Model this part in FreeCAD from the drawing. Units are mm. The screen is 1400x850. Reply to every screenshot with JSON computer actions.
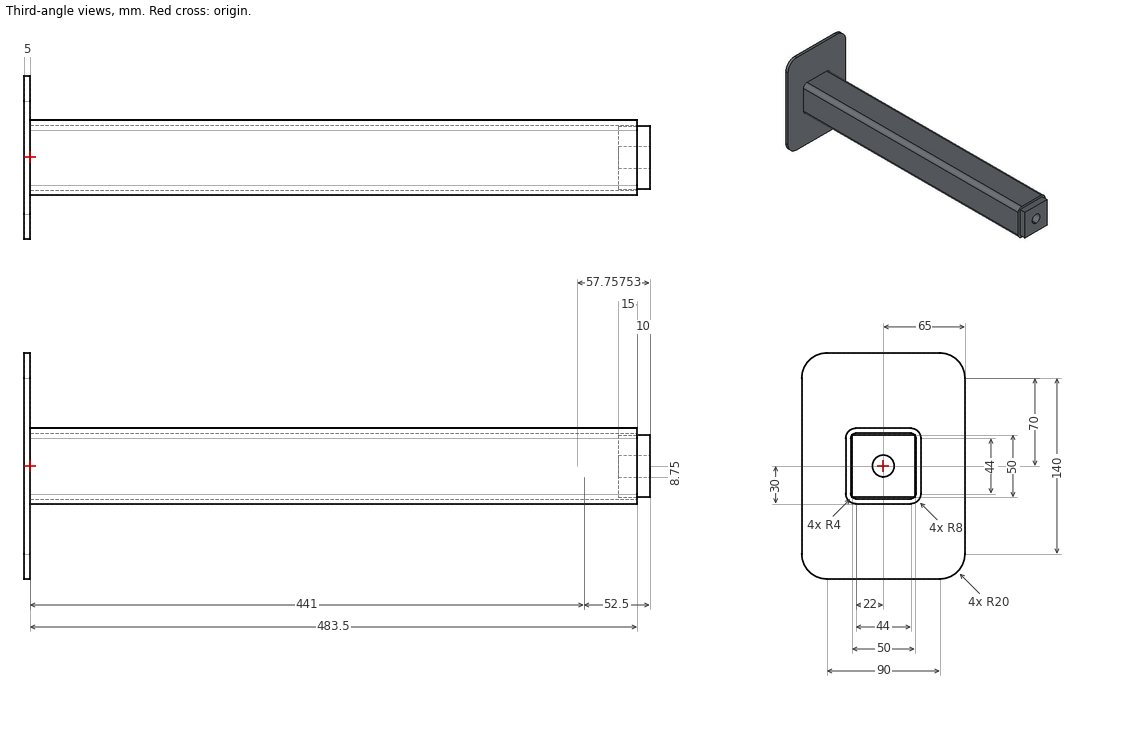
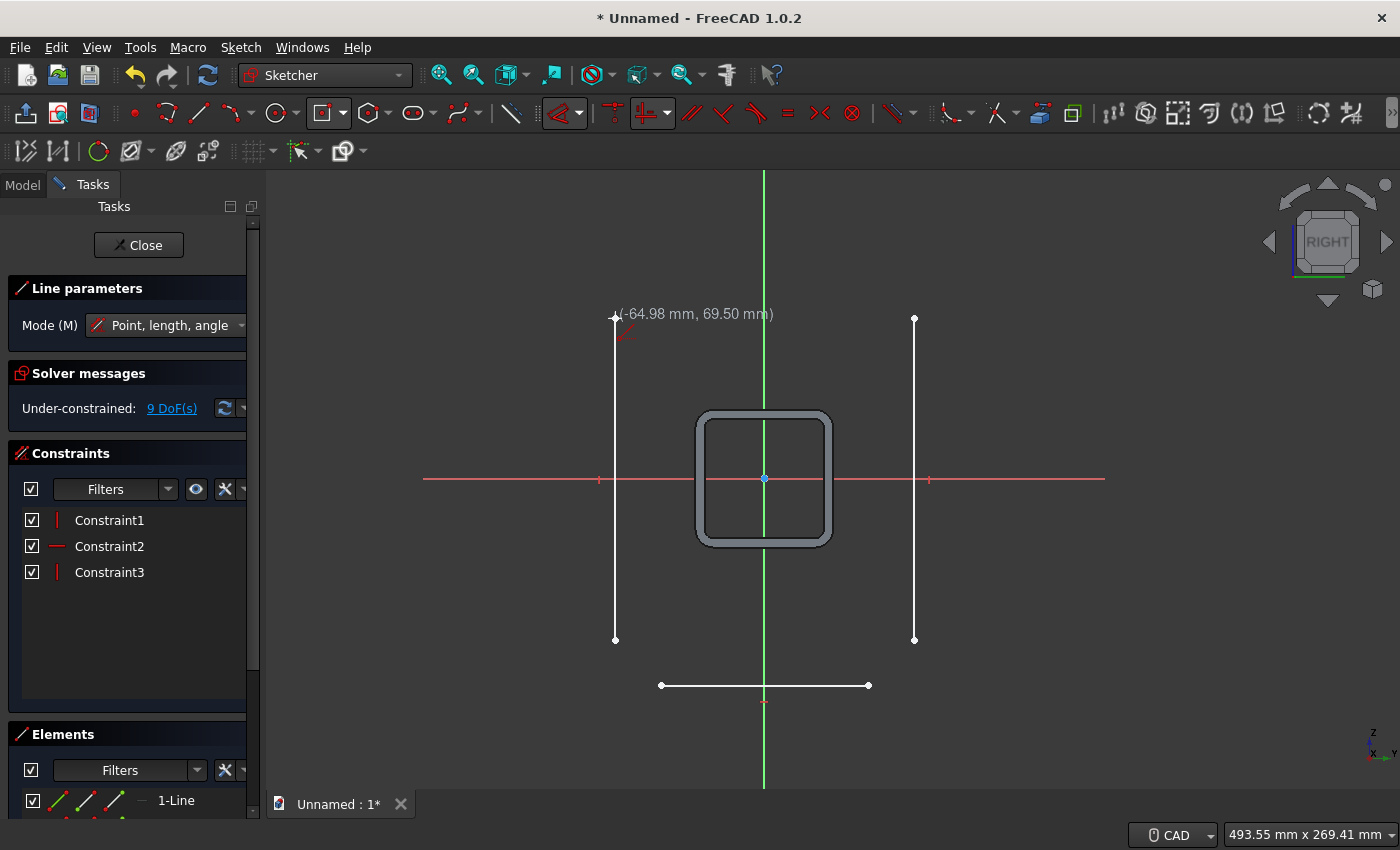
{"action": "left_click", "coordinate": [661, 272]}
{"action": "left_click", "coordinate": [868, 272]}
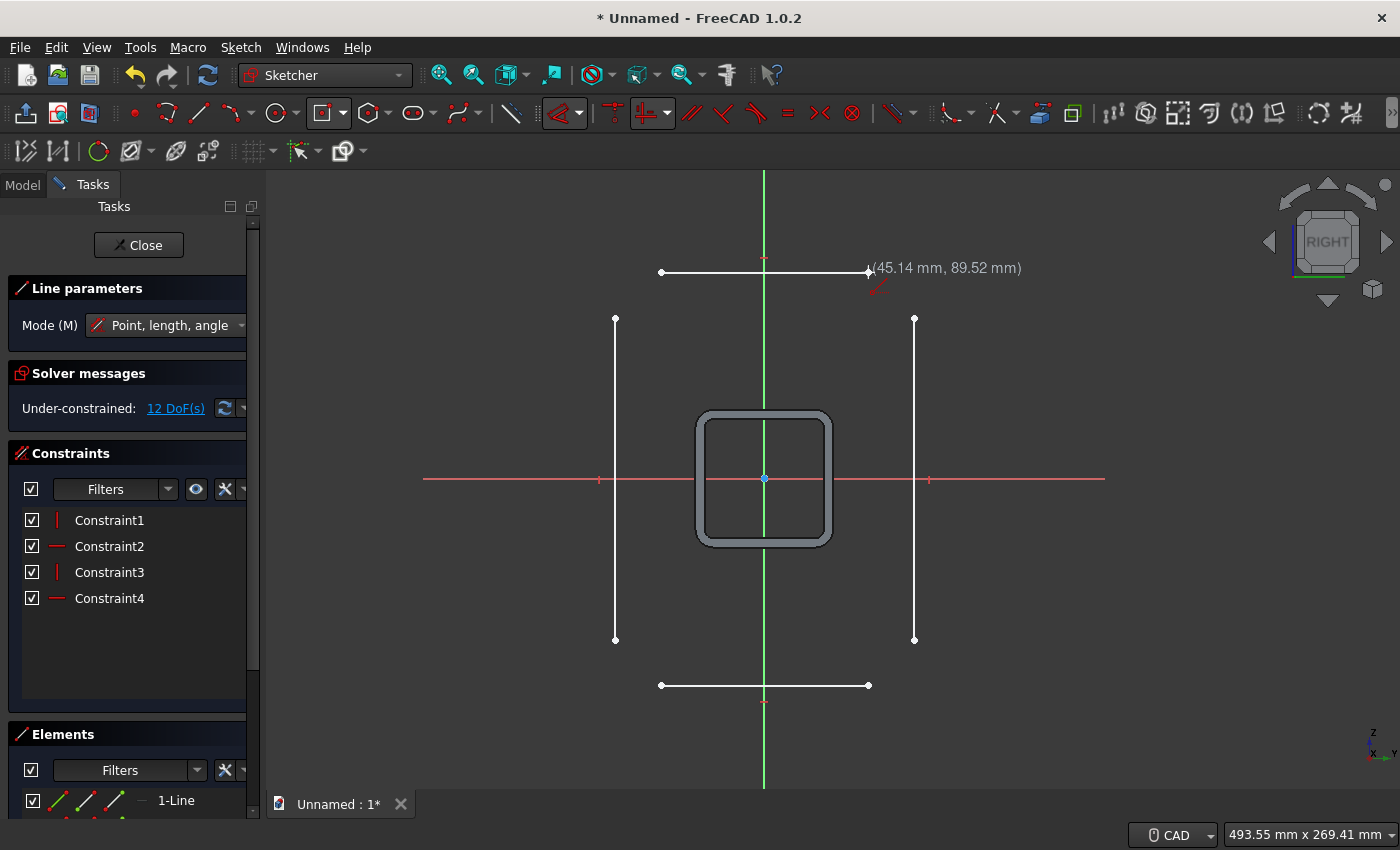
{"action": "left_click", "coordinate": [232, 114]}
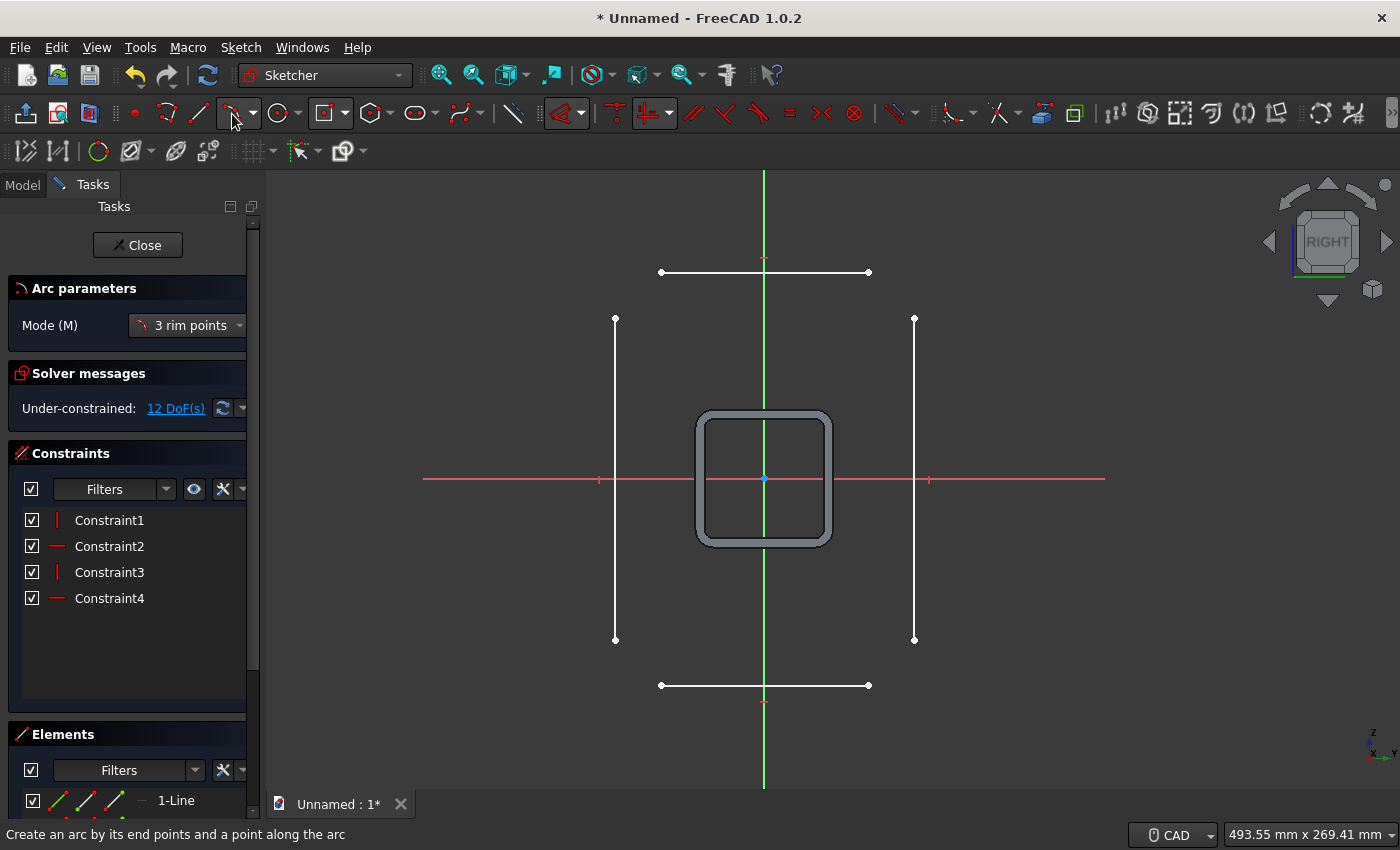
{"action": "left_click", "coordinate": [914, 641]}
{"action": "left_click", "coordinate": [868, 686]}
{"action": "left_click", "coordinate": [900, 672]}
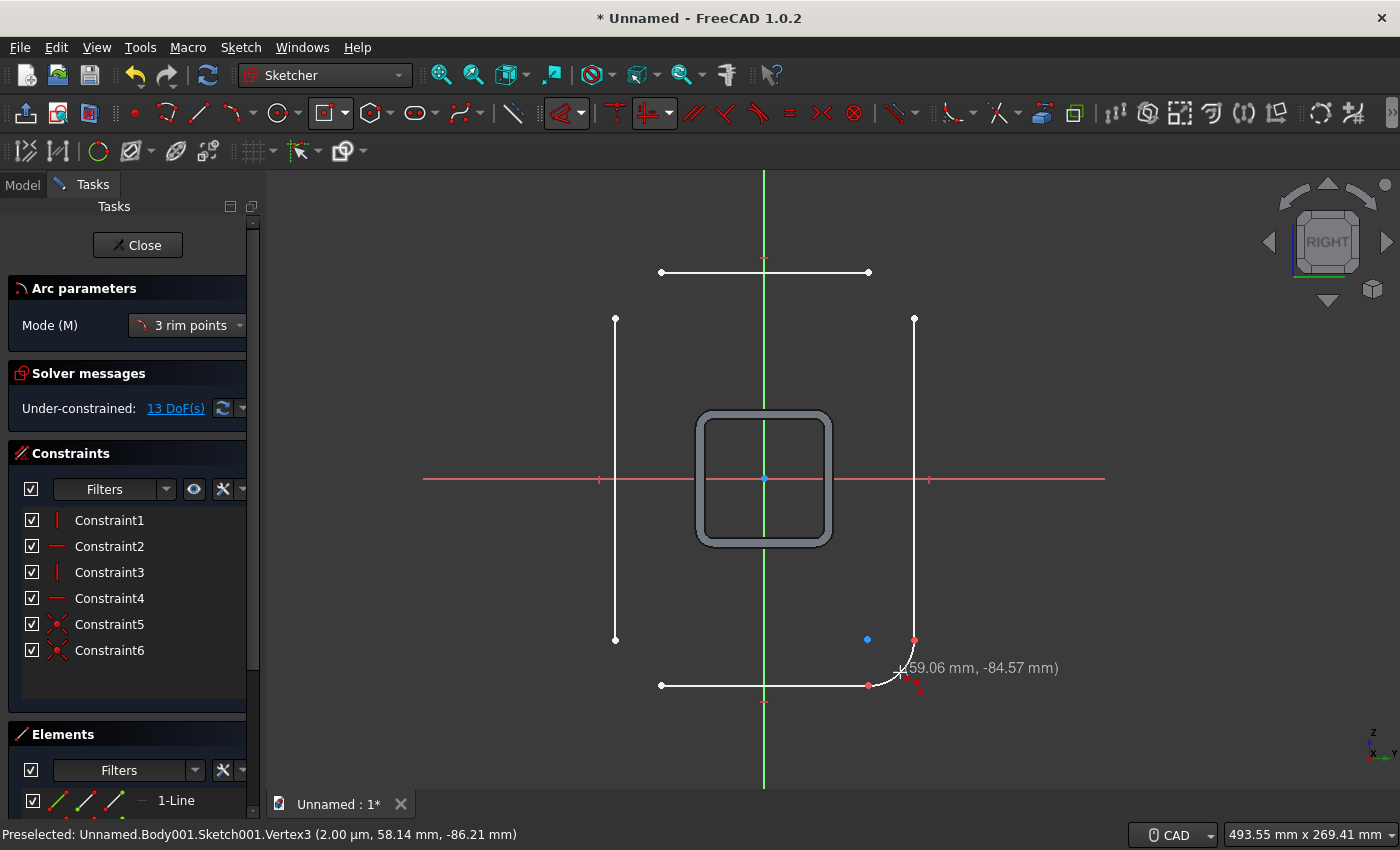
{"action": "left_click", "coordinate": [661, 686]}
{"action": "left_click", "coordinate": [615, 641]}
{"action": "left_click", "coordinate": [628, 672]}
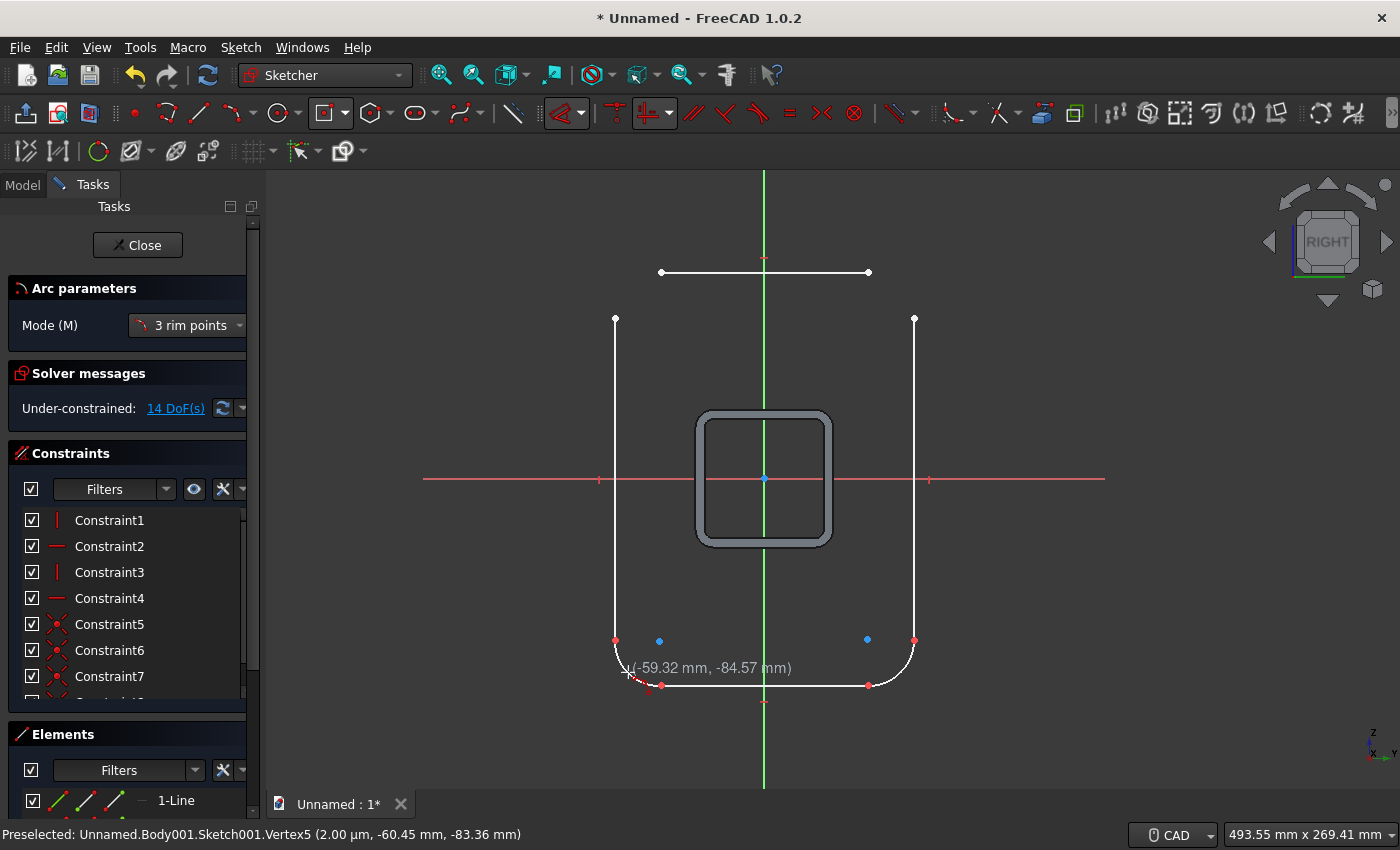
{"action": "left_click", "coordinate": [615, 319]}
{"action": "left_click", "coordinate": [661, 273]}
{"action": "left_click", "coordinate": [628, 285]}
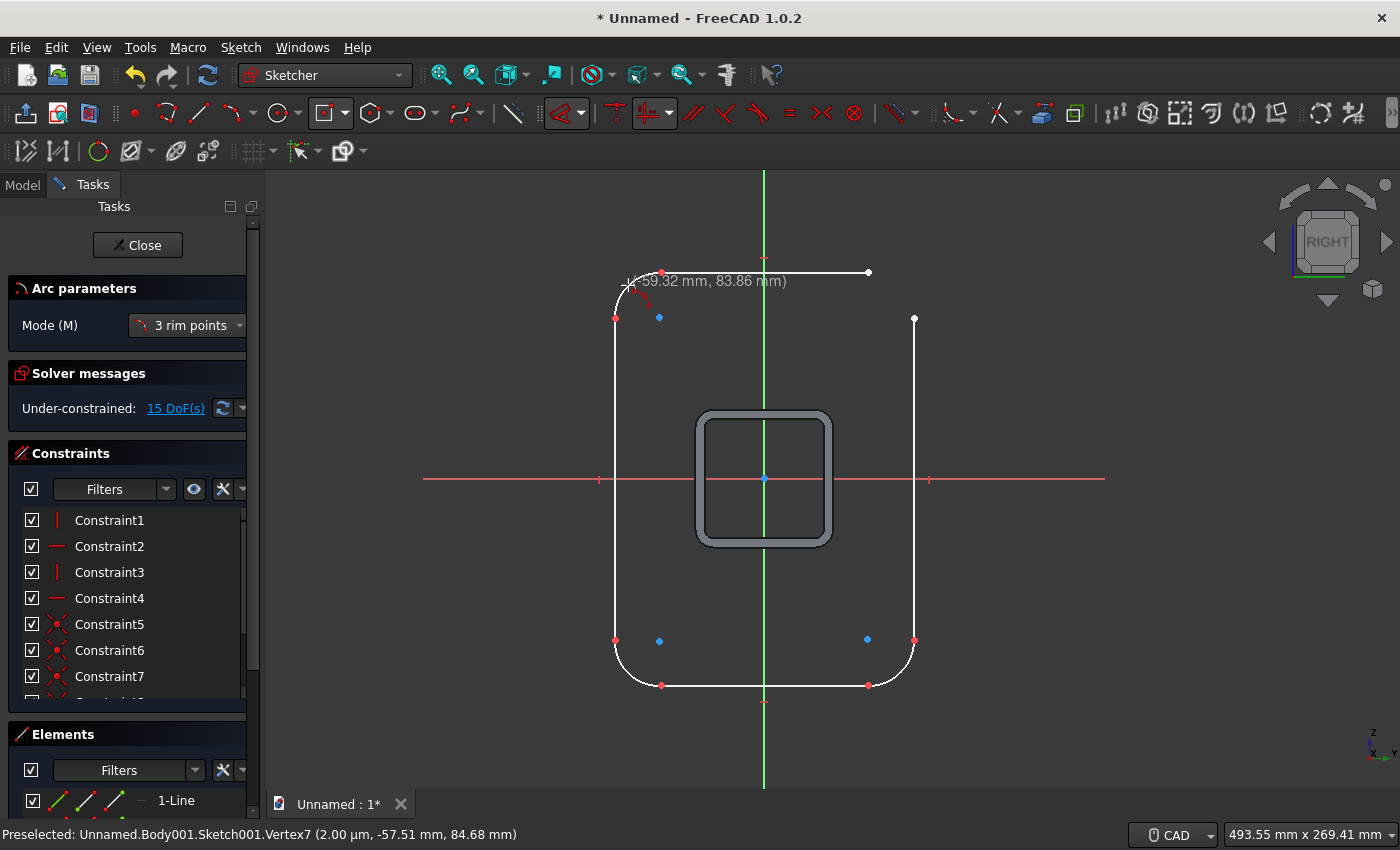
{"action": "left_click", "coordinate": [868, 273]}
{"action": "left_click", "coordinate": [914, 319]}
{"action": "left_click", "coordinate": [900, 285]}
{"action": "key", "text": "Escape"}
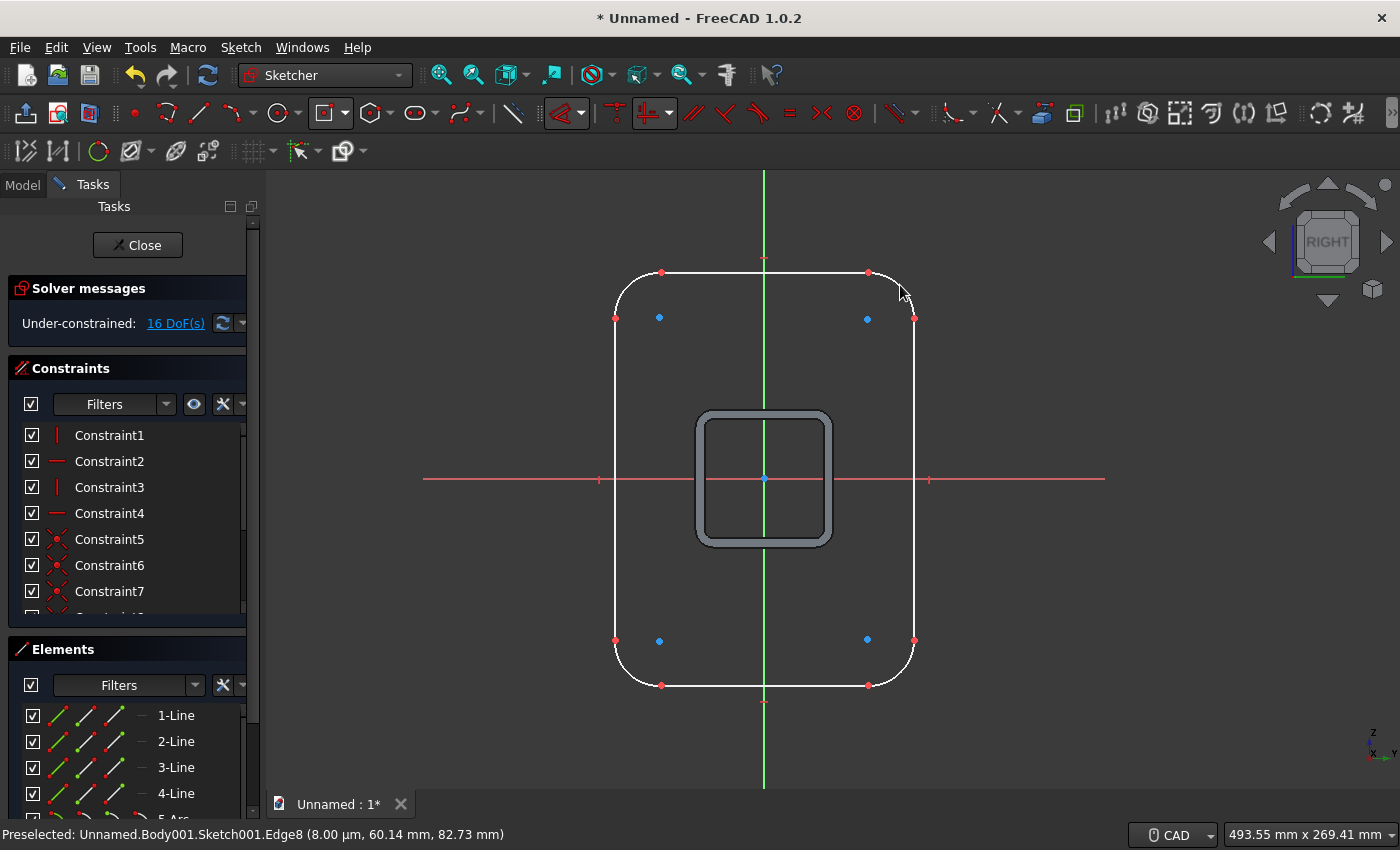
{"action": "left_click", "coordinate": [914, 416]}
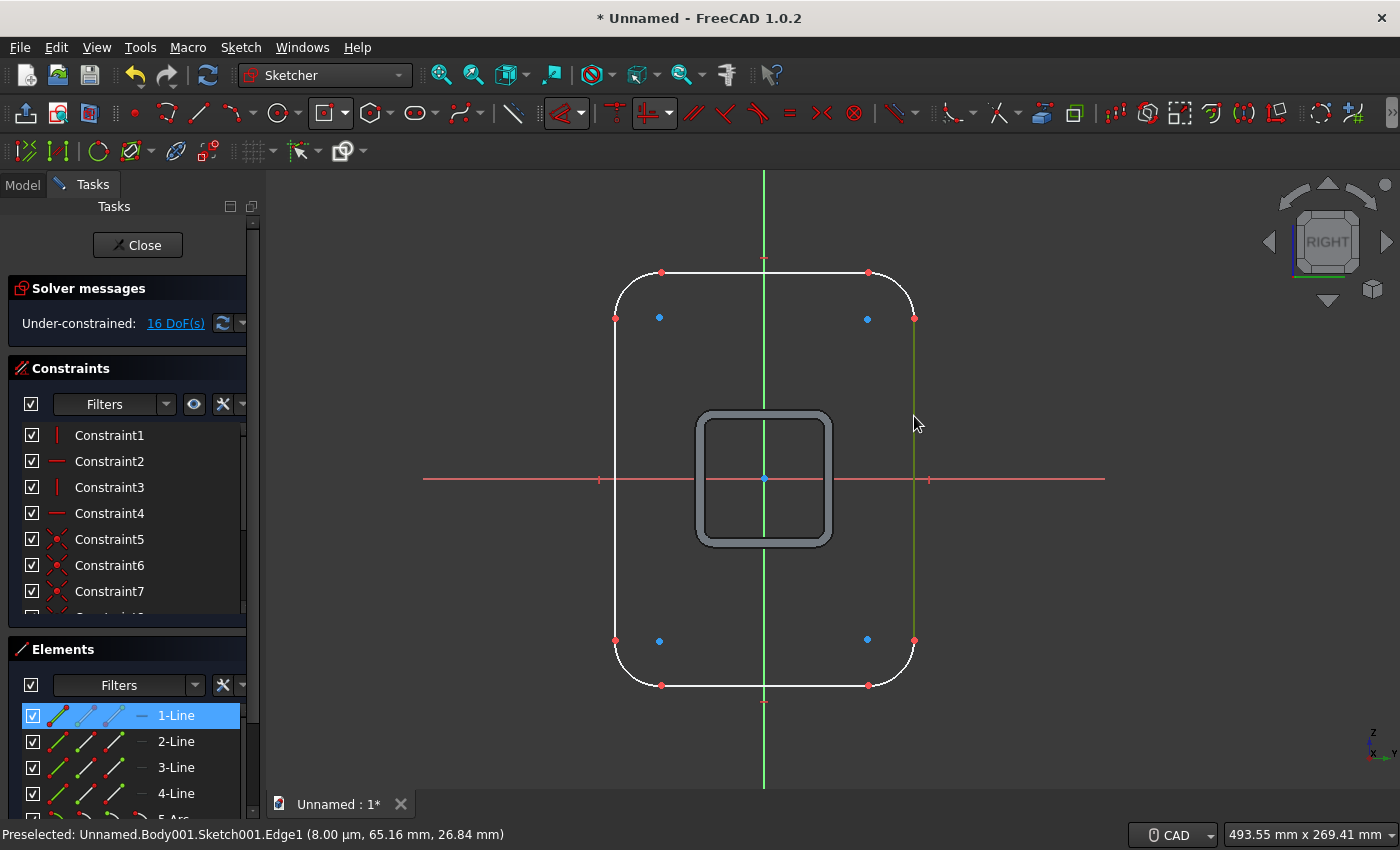
{"action": "left_click", "coordinate": [889, 681]}